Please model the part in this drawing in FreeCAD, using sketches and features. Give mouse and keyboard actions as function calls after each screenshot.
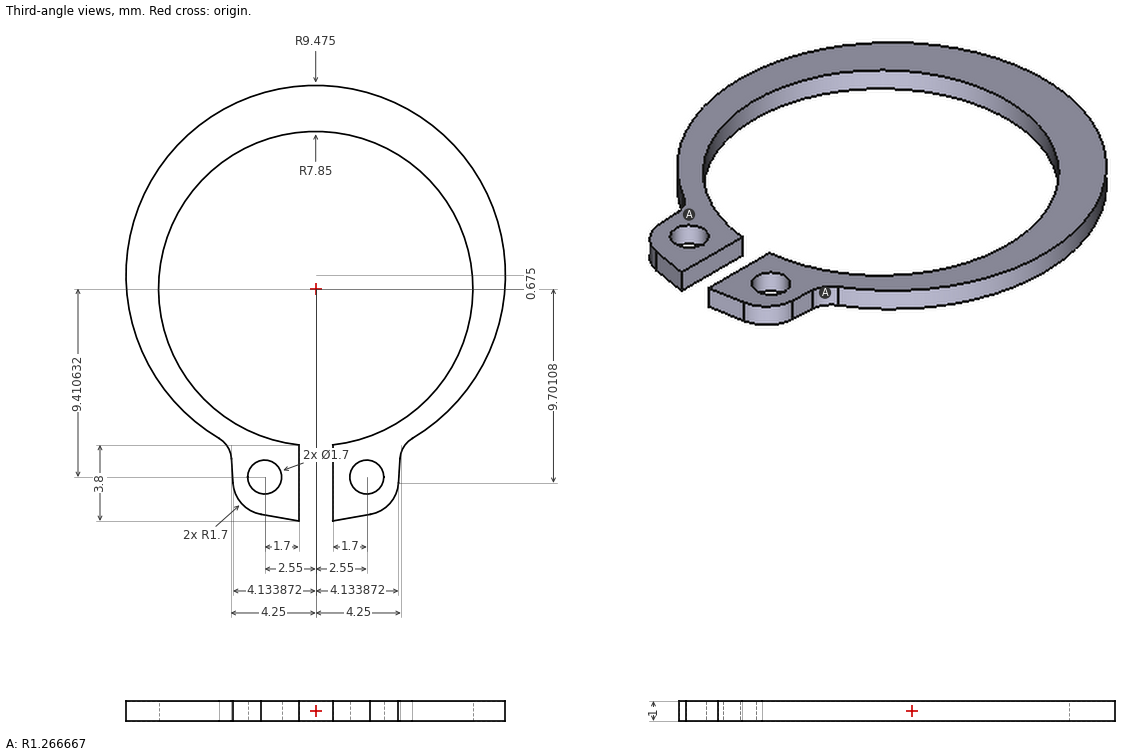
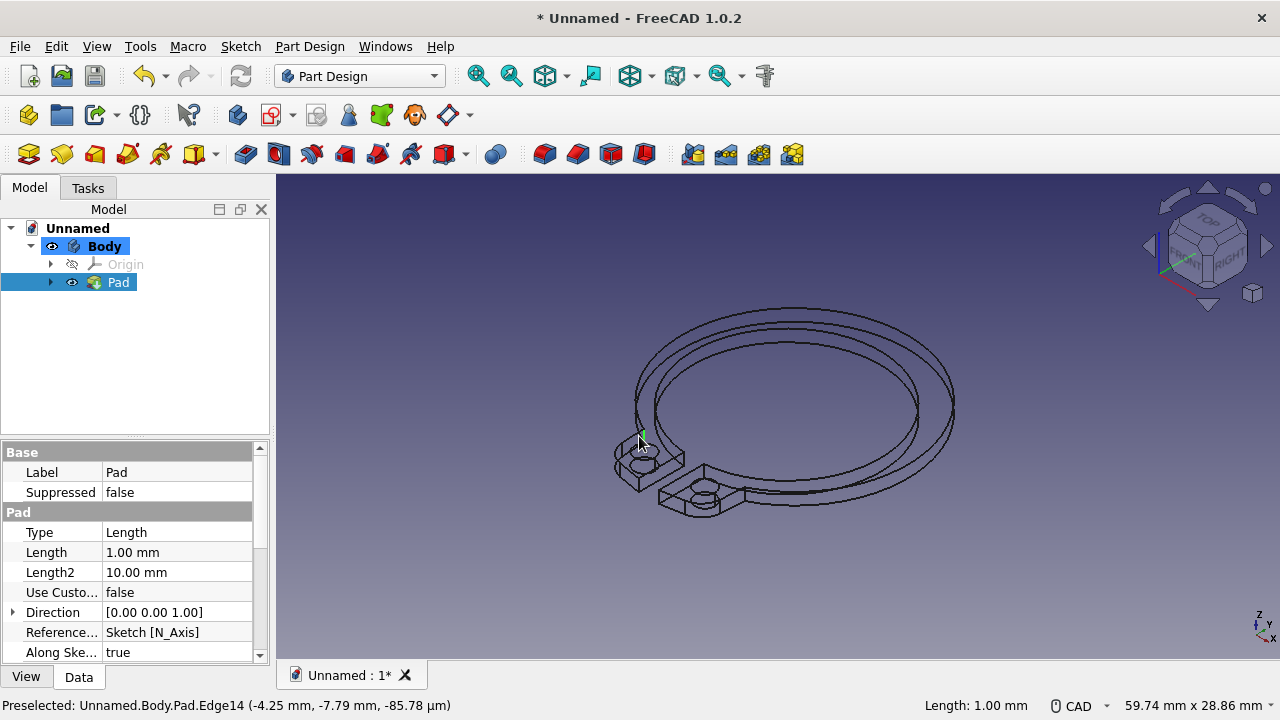
click(745, 495, ctrl)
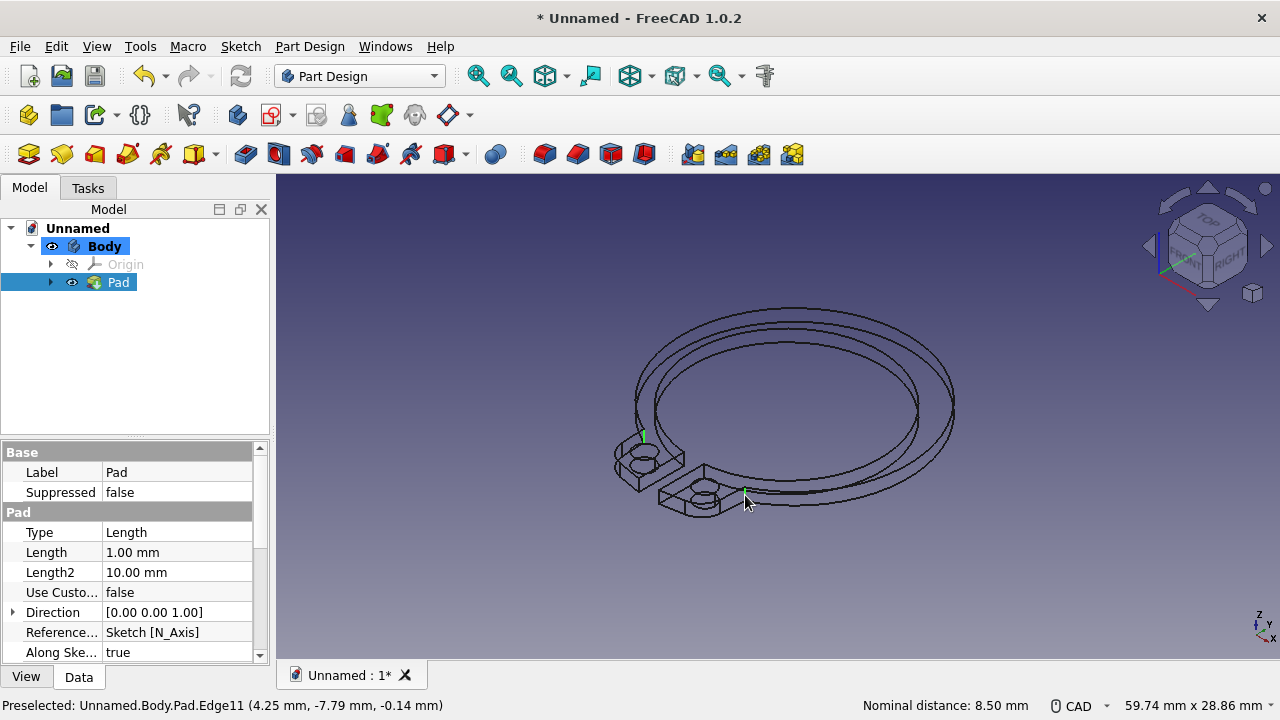
key(v)
key(1)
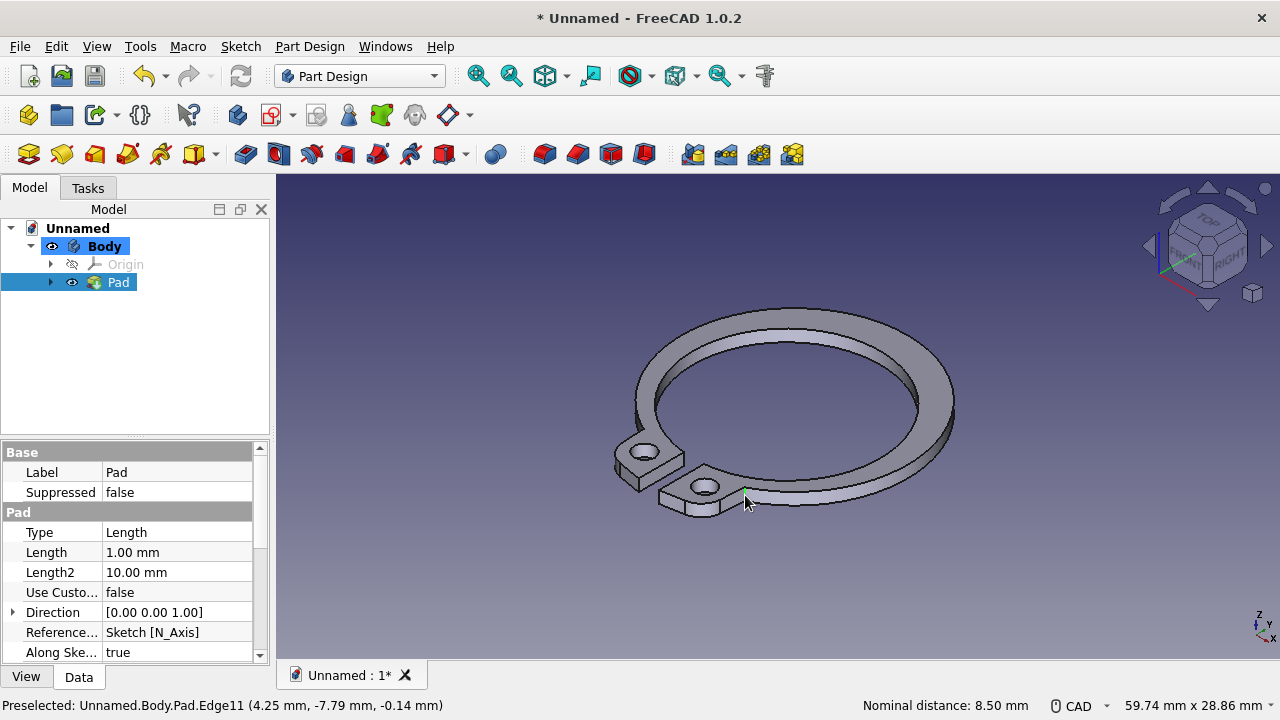
click(545, 154)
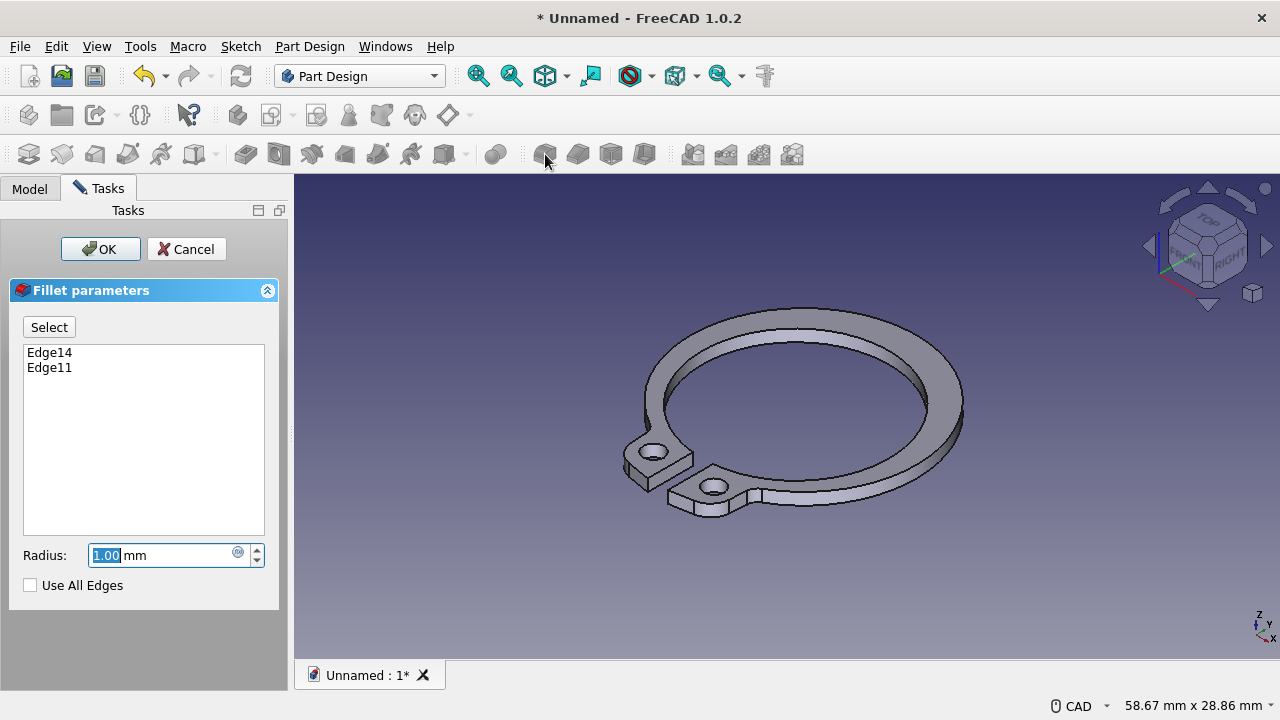
text(1.266667)
key(Tab)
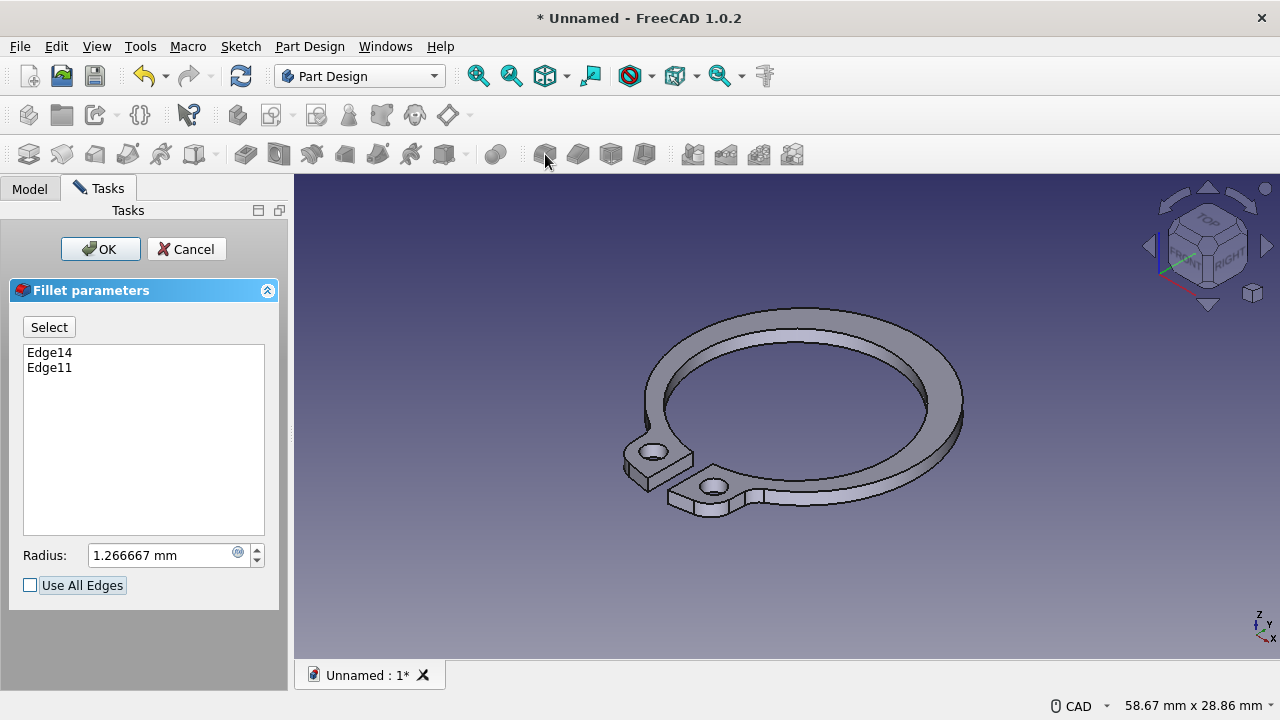
click(101, 249)